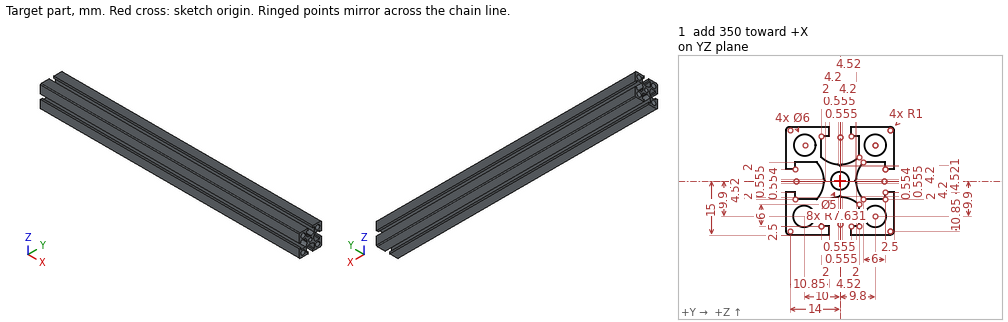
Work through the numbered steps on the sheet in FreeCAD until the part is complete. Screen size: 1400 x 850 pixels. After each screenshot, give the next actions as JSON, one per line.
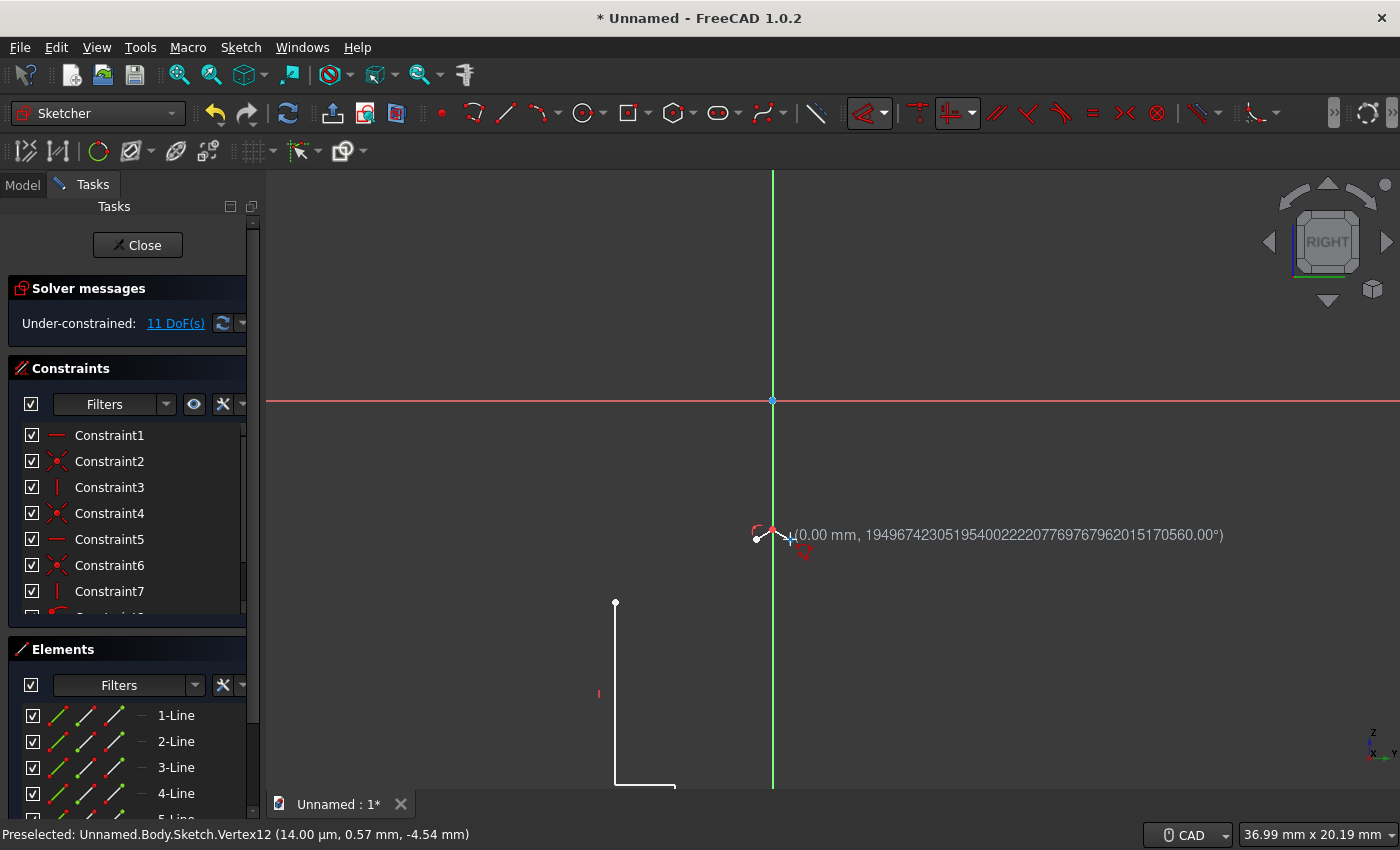
{"action": "left_click", "coordinate": [930, 600]}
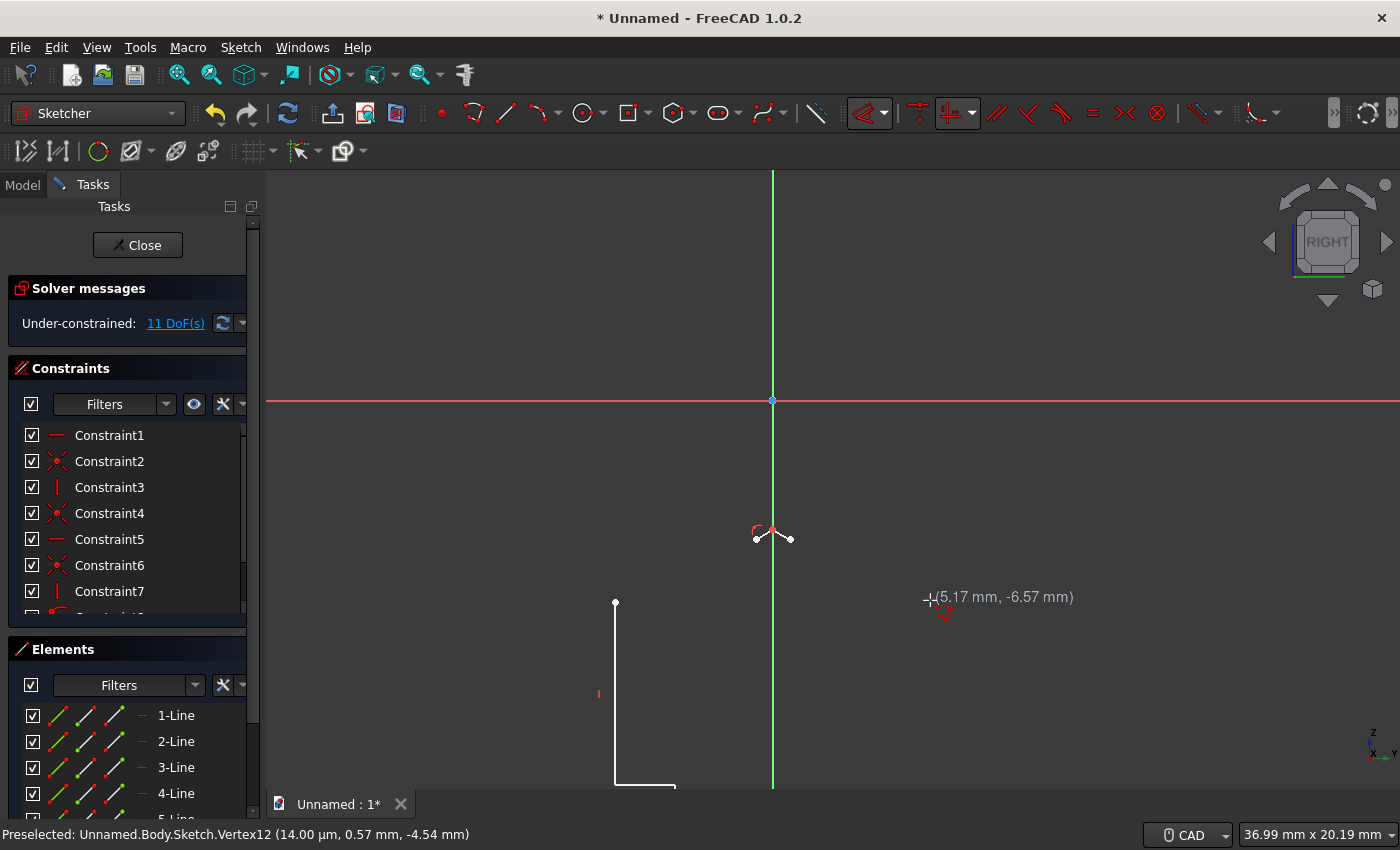
{"action": "scroll", "coordinate": [758, 544], "scroll_direction": "down", "scroll_amount": 4}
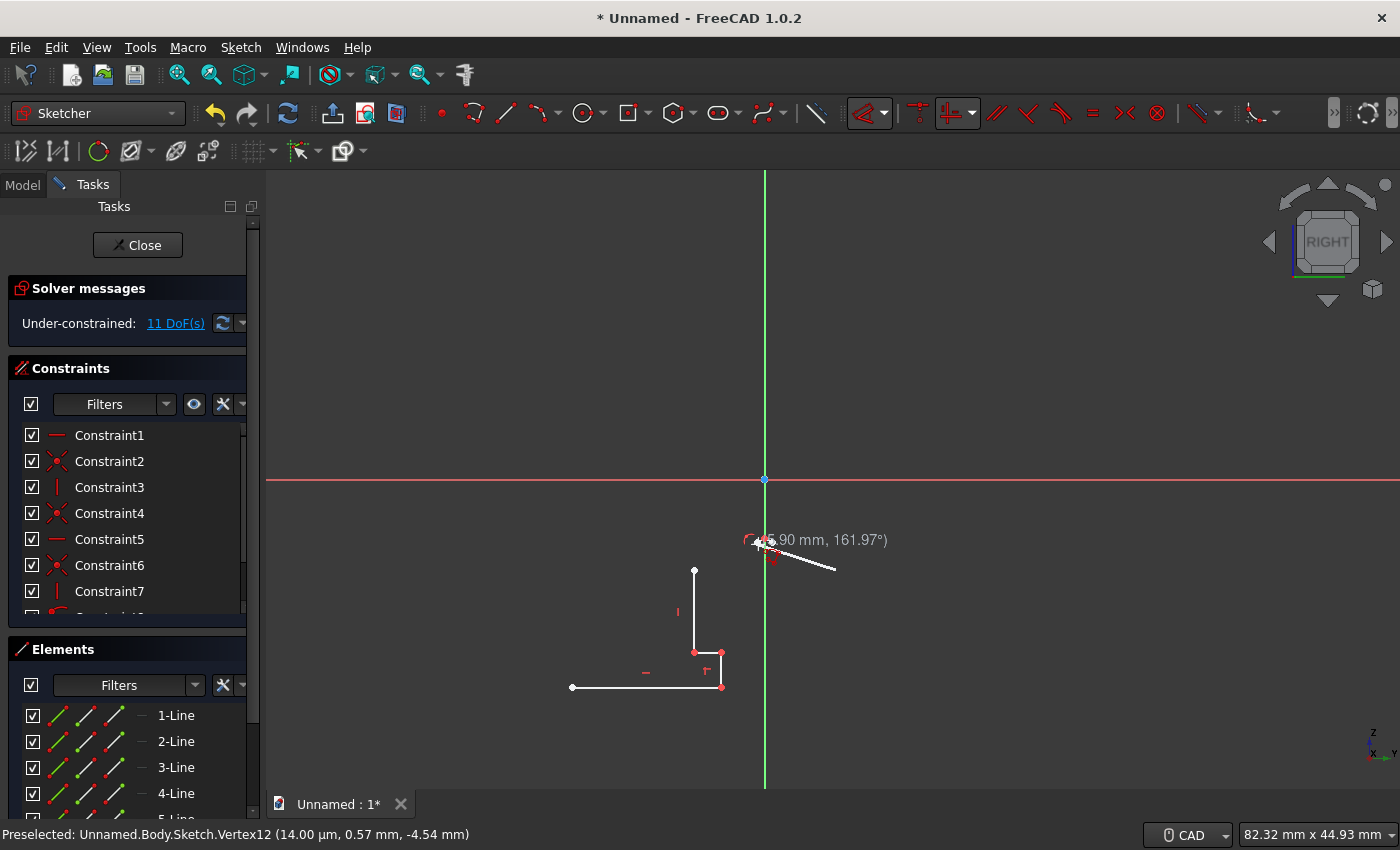
{"action": "left_click", "coordinate": [836, 652]}
{"action": "left_click", "coordinate": [808, 652]}
{"action": "left_click", "coordinate": [808, 687]}
{"action": "left_click", "coordinate": [958, 687]}
{"action": "right_click", "coordinate": [958, 687]}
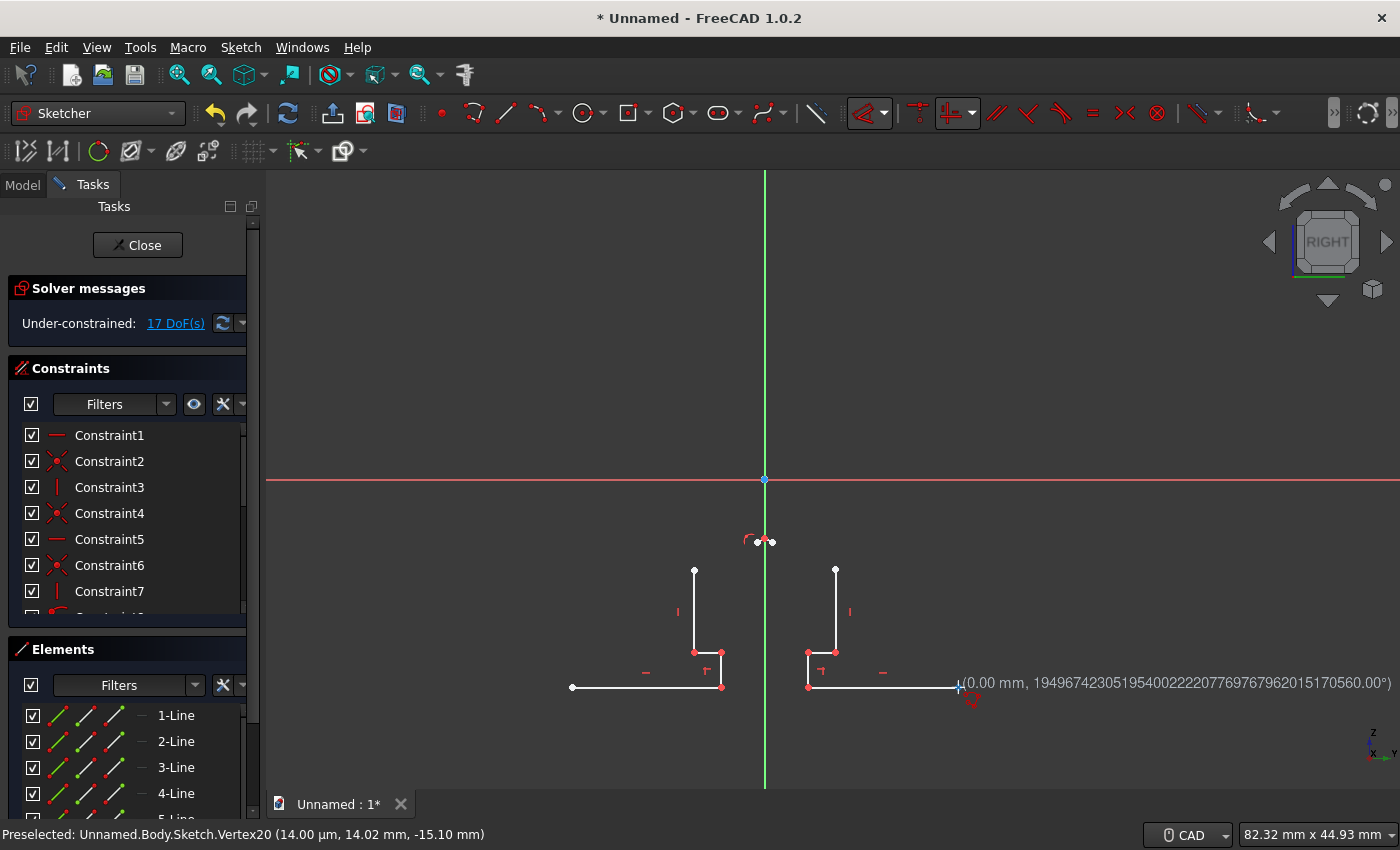
{"action": "left_click", "coordinate": [971, 673]}
{"action": "left_click", "coordinate": [971, 523]}
{"action": "left_click", "coordinate": [937, 523]}
{"action": "left_click", "coordinate": [937, 551]}
{"action": "left_click", "coordinate": [854, 551]}
{"action": "right_click", "coordinate": [854, 551]}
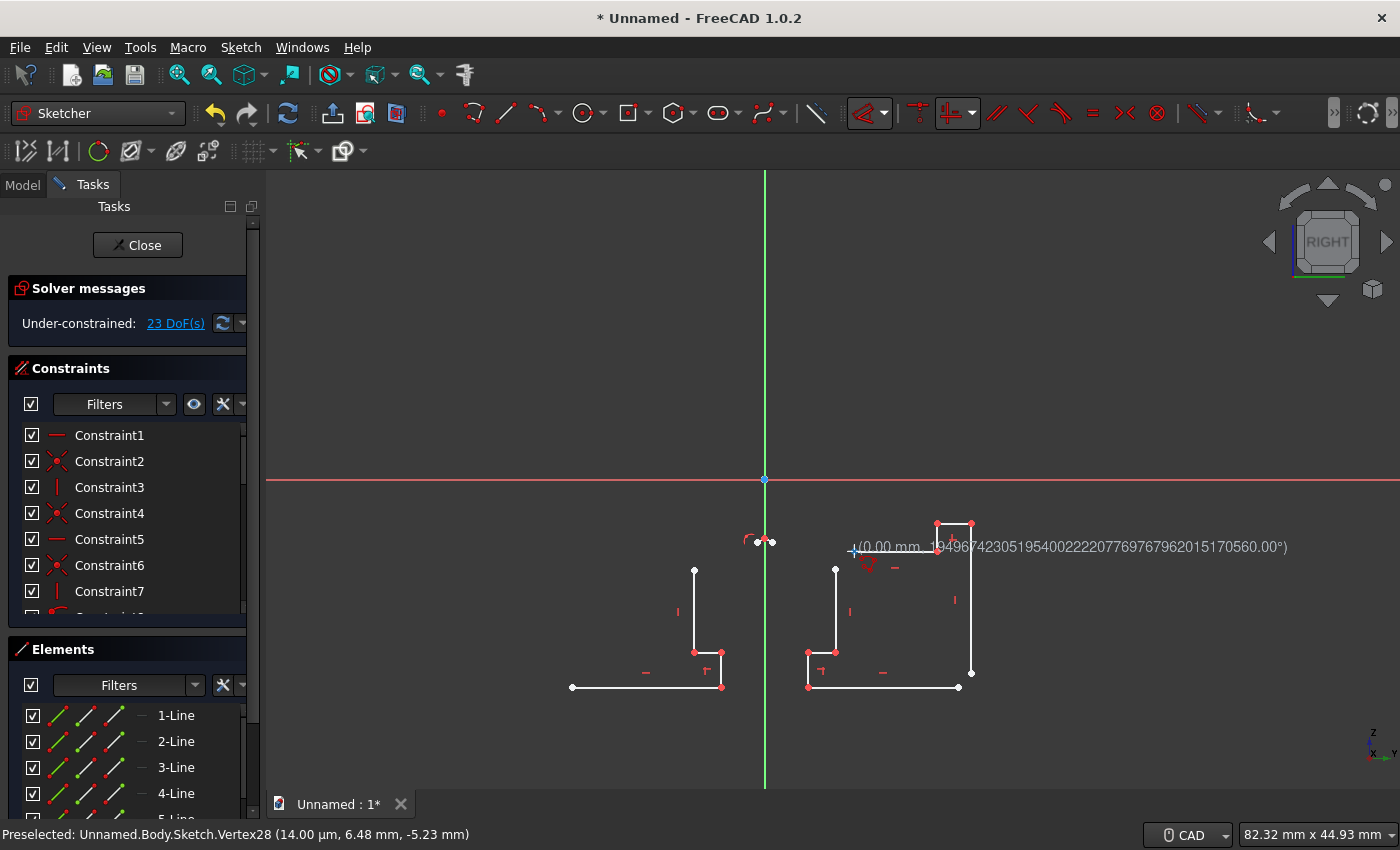
{"action": "scroll", "coordinate": [827, 488], "scroll_direction": "up", "scroll_amount": 4}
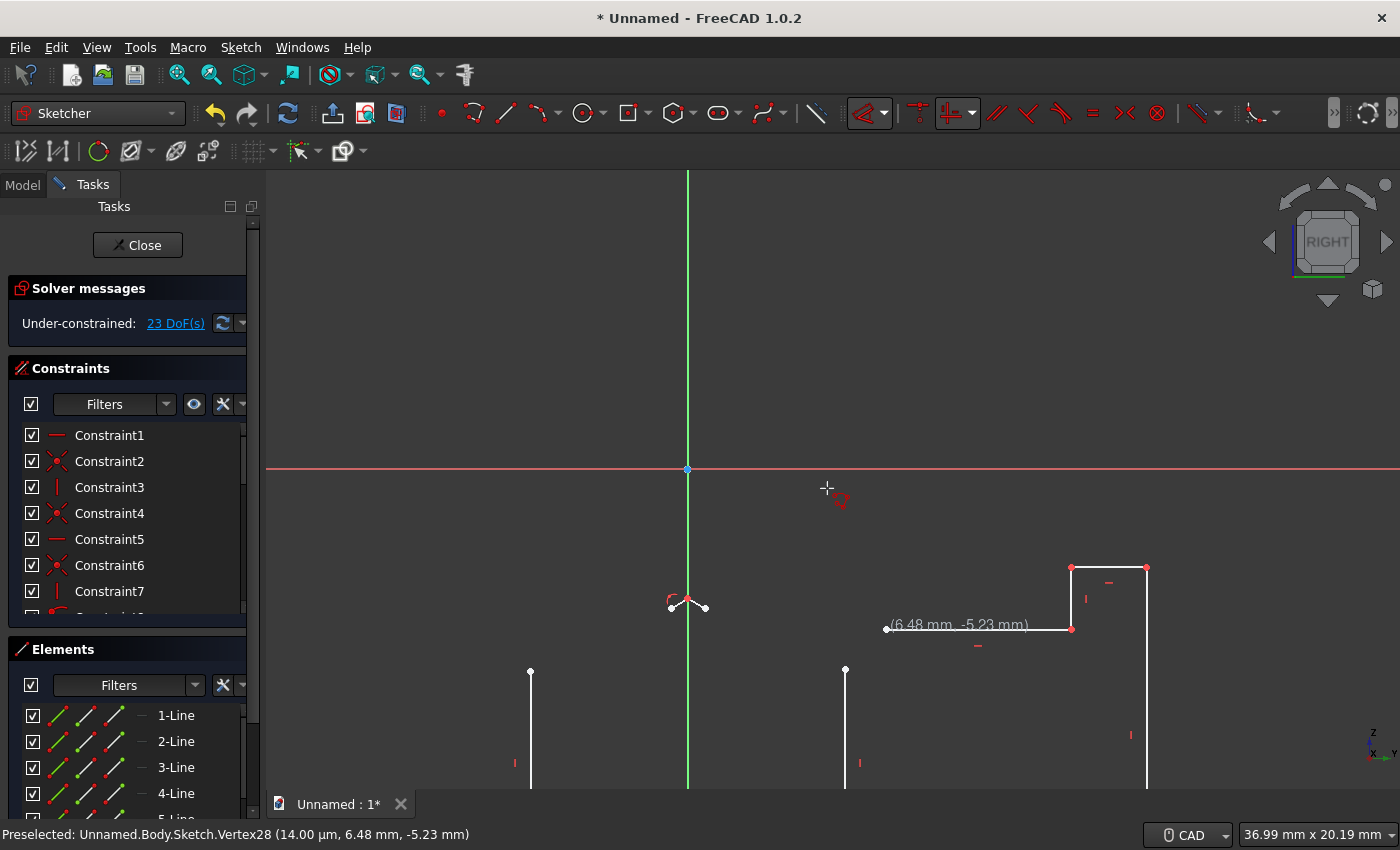
{"action": "left_click", "coordinate": [827, 486]}
{"action": "left_click", "coordinate": [817, 469]}
{"action": "left_click", "coordinate": [827, 452]}
{"action": "right_click", "coordinate": [827, 452]}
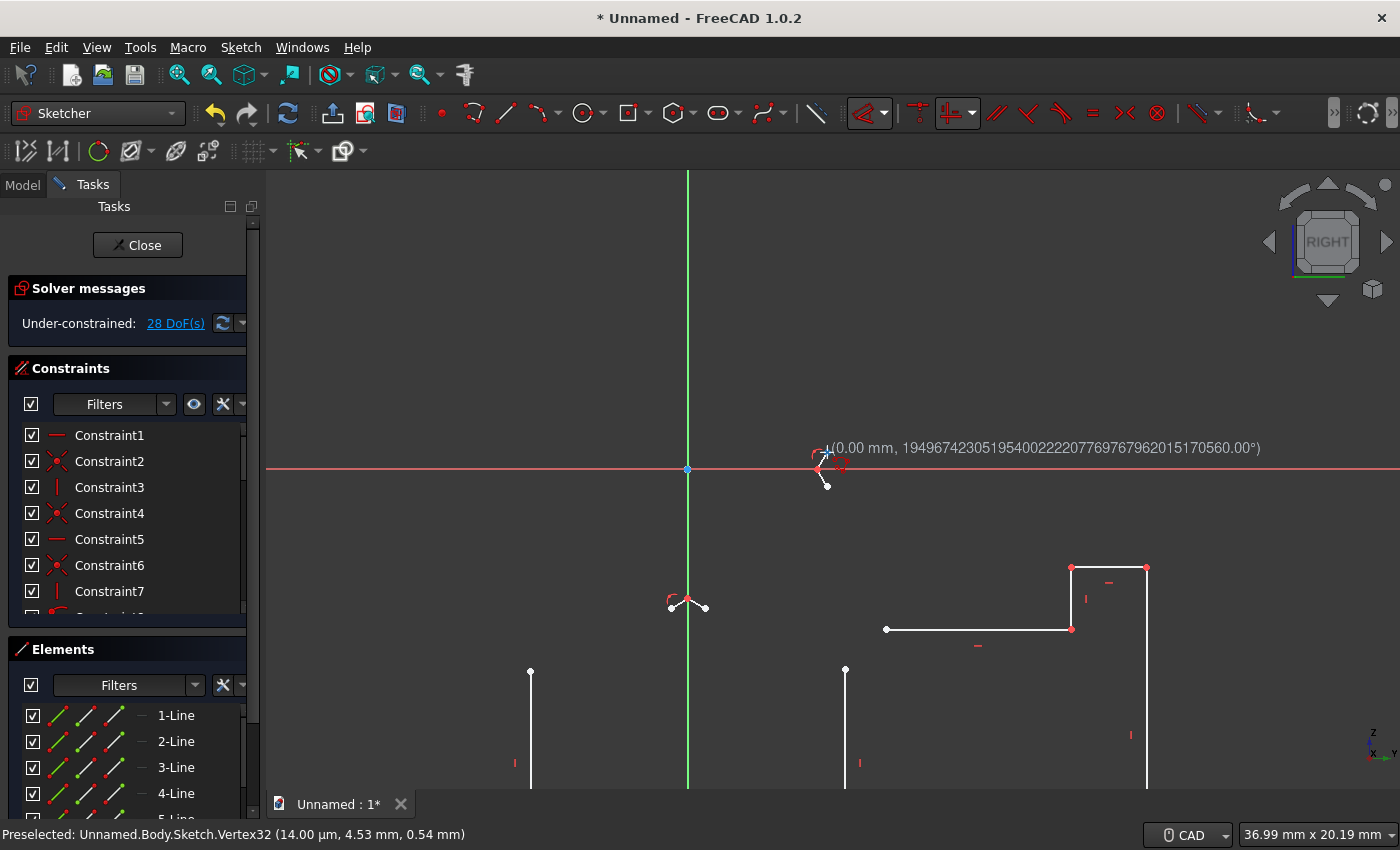
{"action": "left_click", "coordinate": [887, 312]}
{"action": "left_click", "coordinate": [1071, 312]}
{"action": "left_click", "coordinate": [1071, 373]}
{"action": "left_click", "coordinate": [1148, 373]}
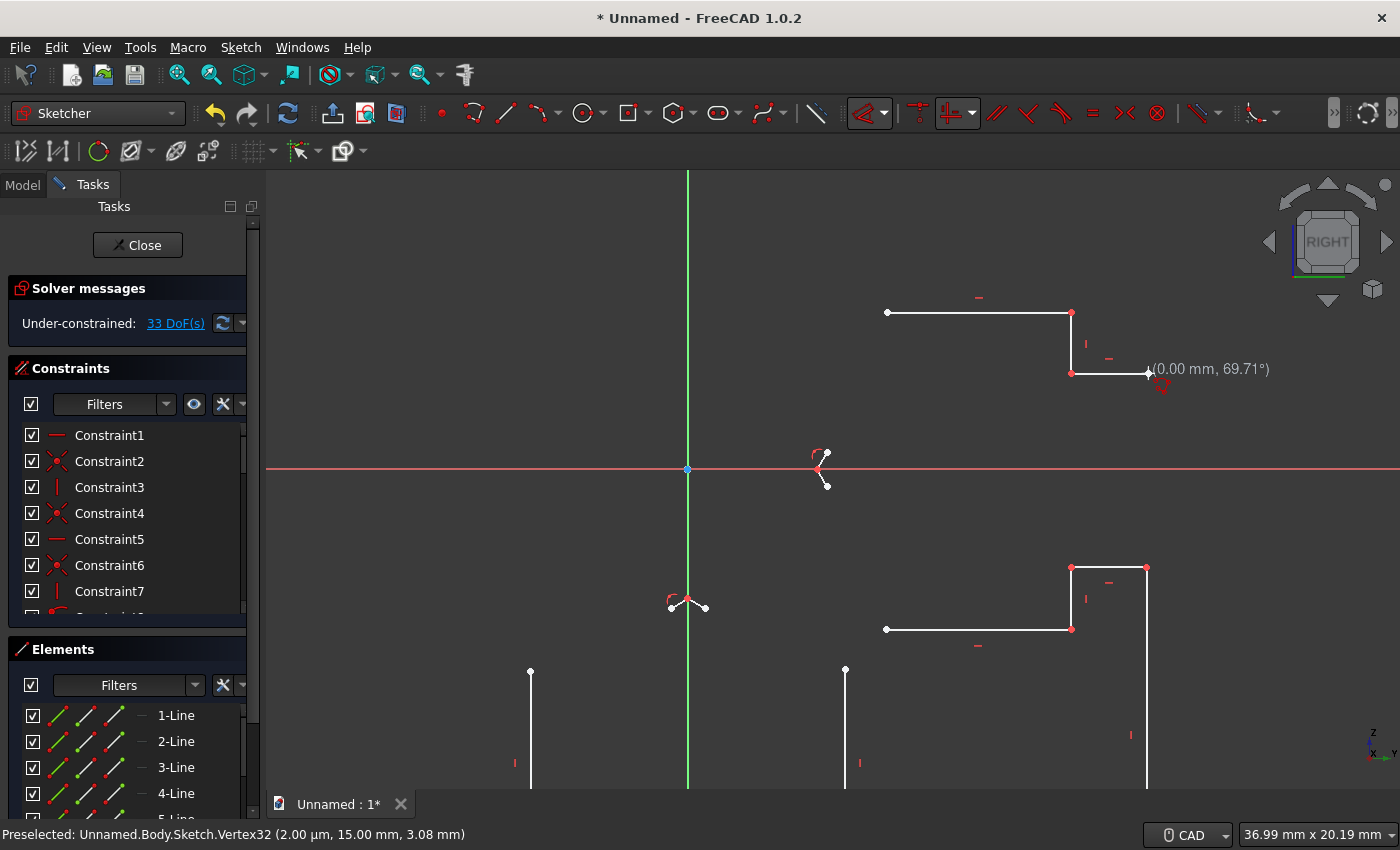
{"action": "scroll", "coordinate": [827, 488], "scroll_direction": "down", "scroll_amount": 4}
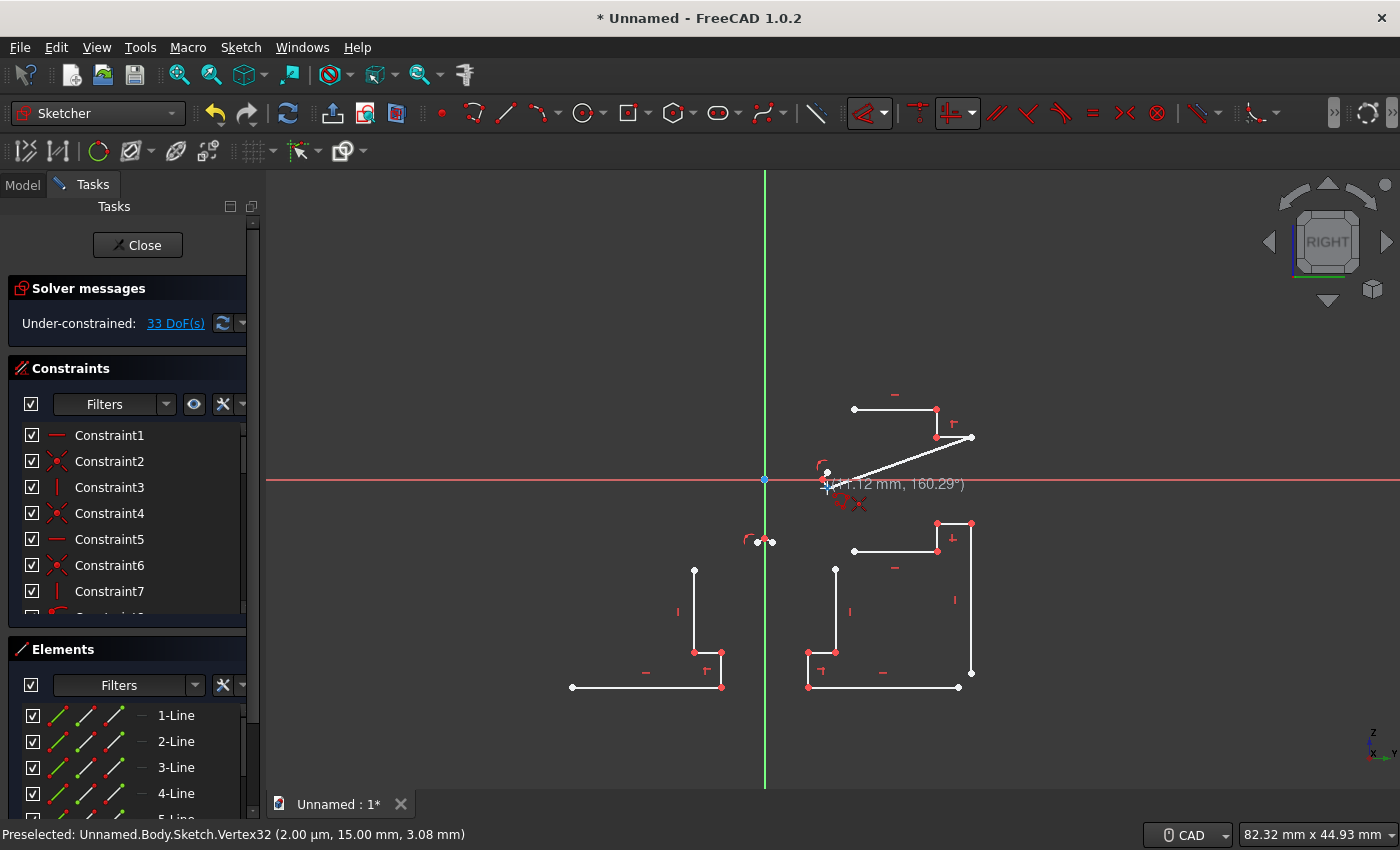
{"action": "left_click", "coordinate": [972, 287]}
{"action": "right_click", "coordinate": [972, 287]}